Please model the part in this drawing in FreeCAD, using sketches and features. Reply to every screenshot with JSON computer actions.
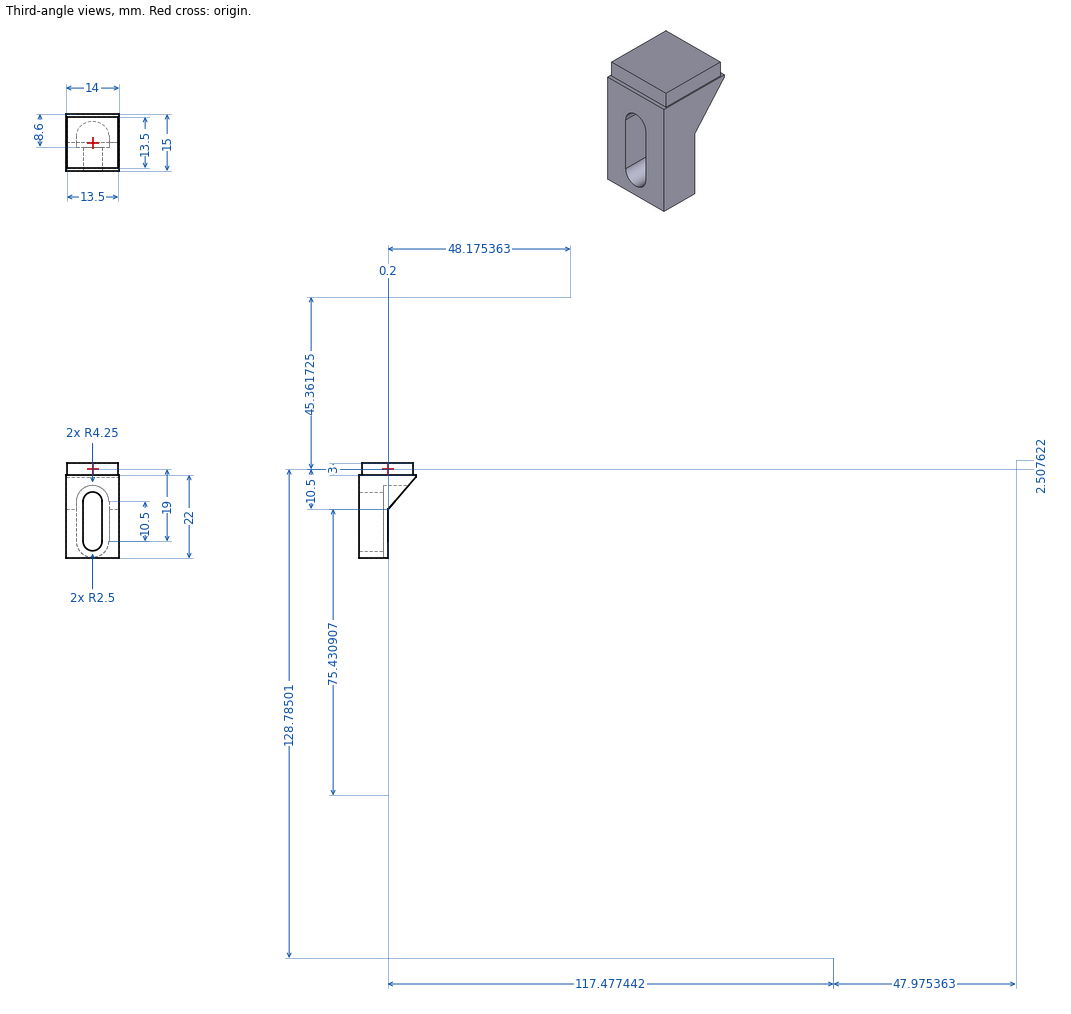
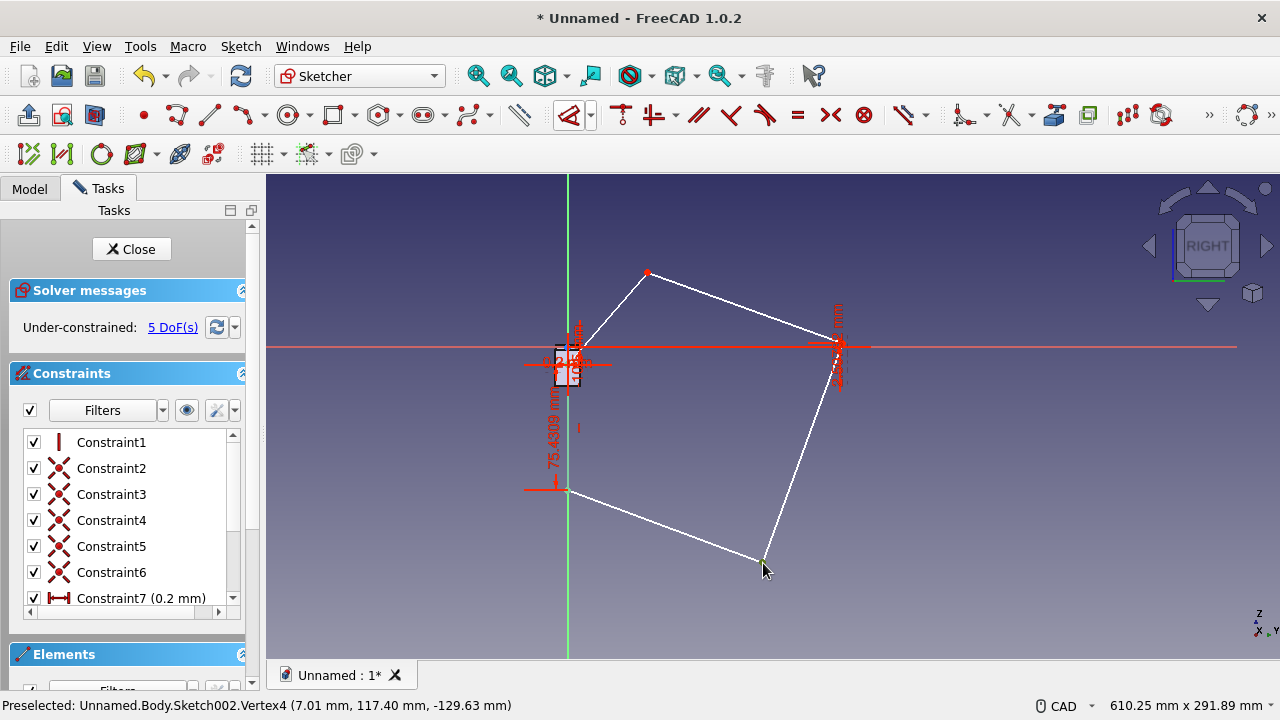
{"action": "key", "text": "i"}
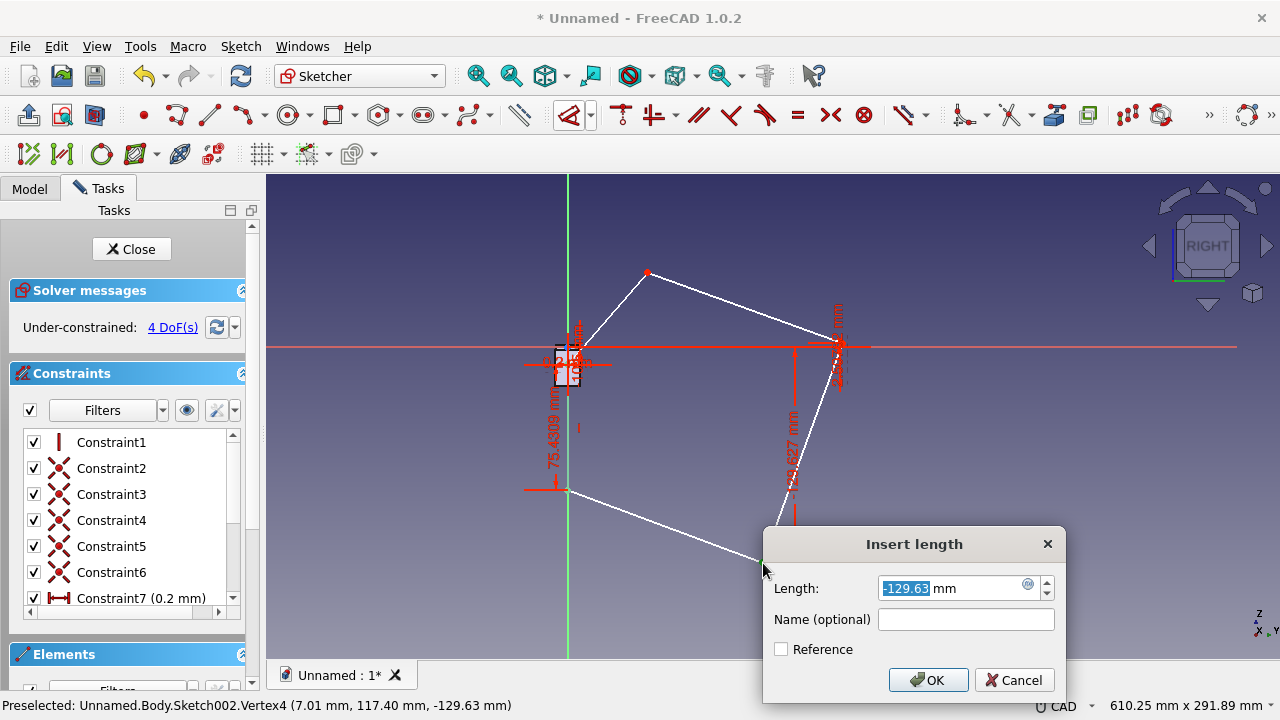
{"action": "type", "text": "-128.78501"}
{"action": "key", "text": "Return"}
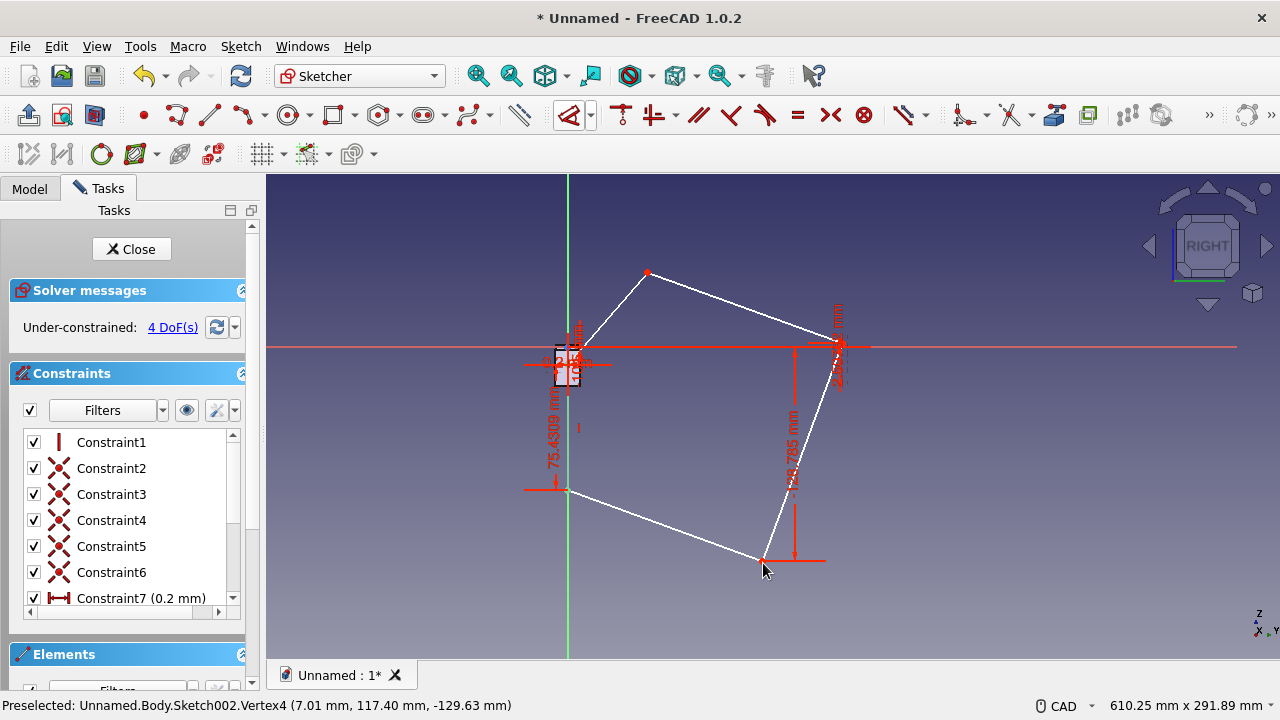
{"action": "left_click", "coordinate": [648, 273]}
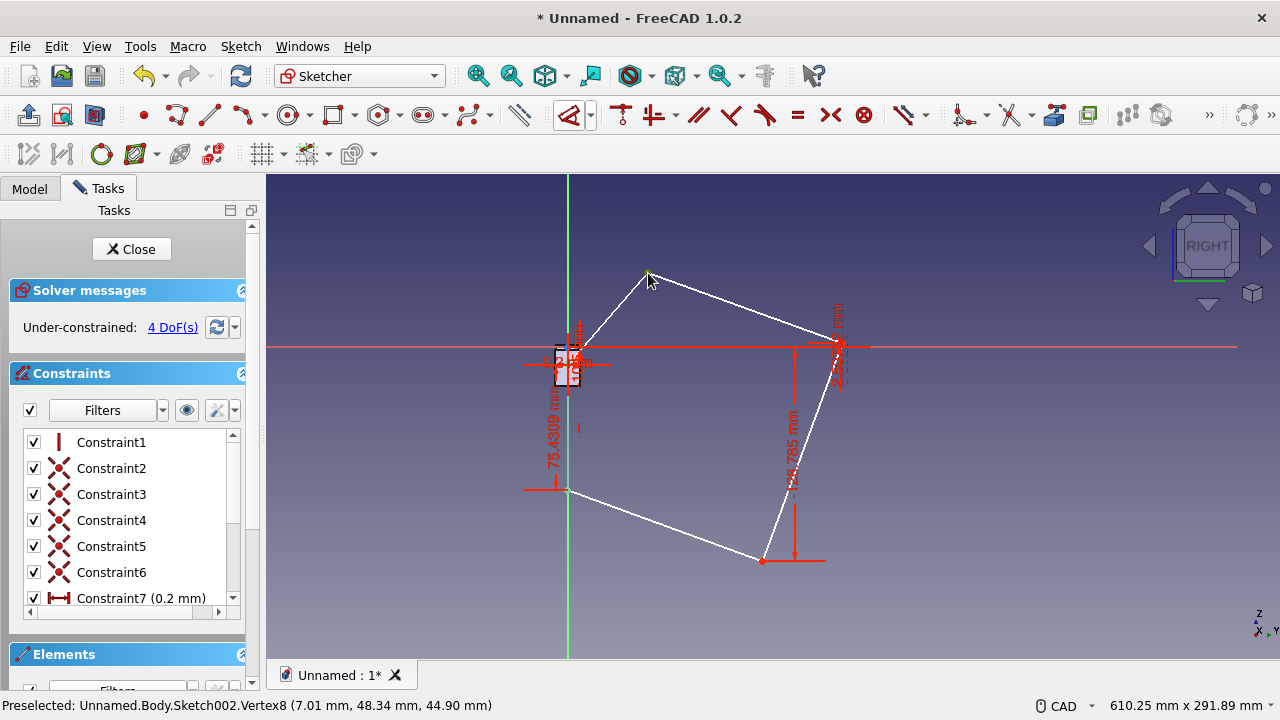
{"action": "key", "text": "l"}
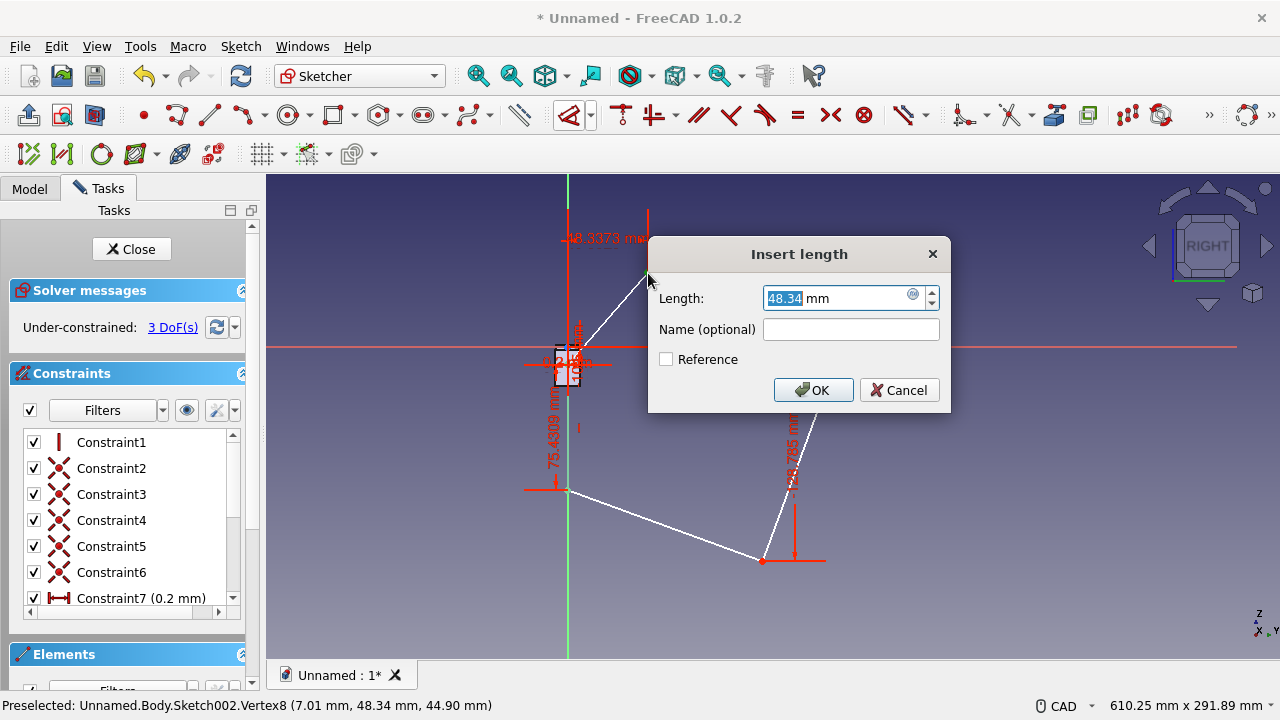
{"action": "type", "text": "48.175363"}
{"action": "key", "text": "Return"}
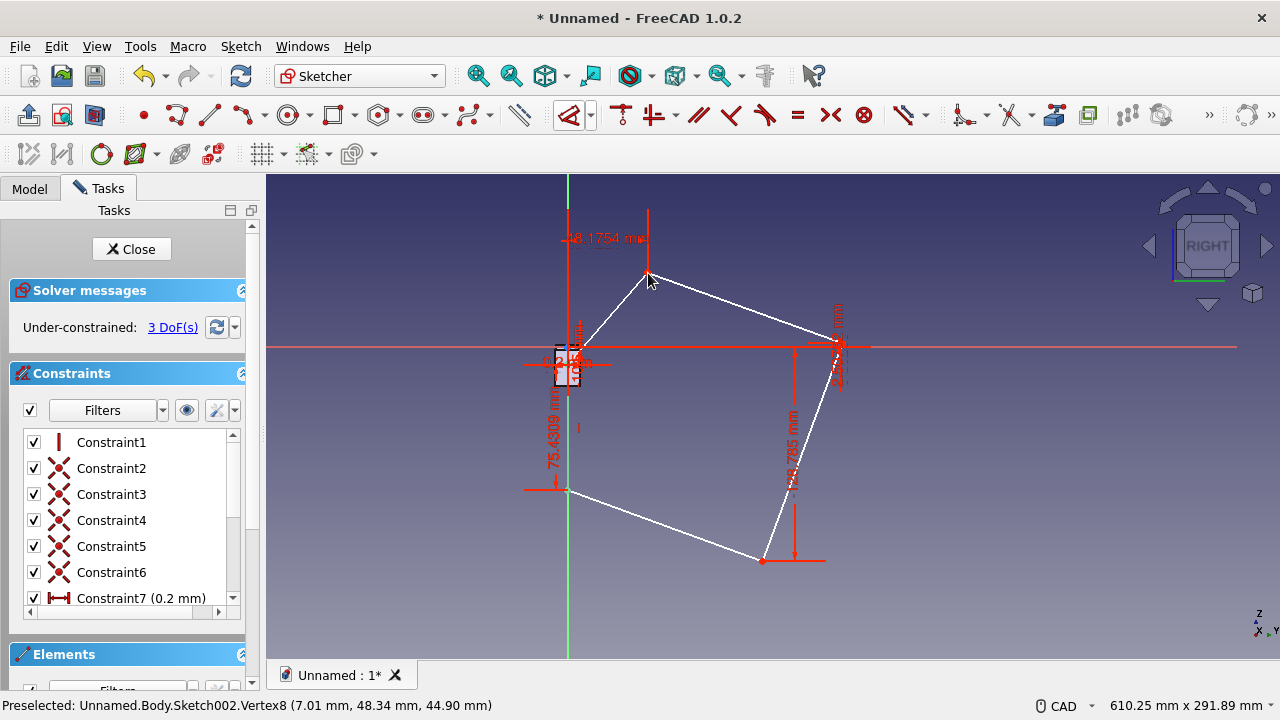
{"action": "left_click", "coordinate": [648, 273]}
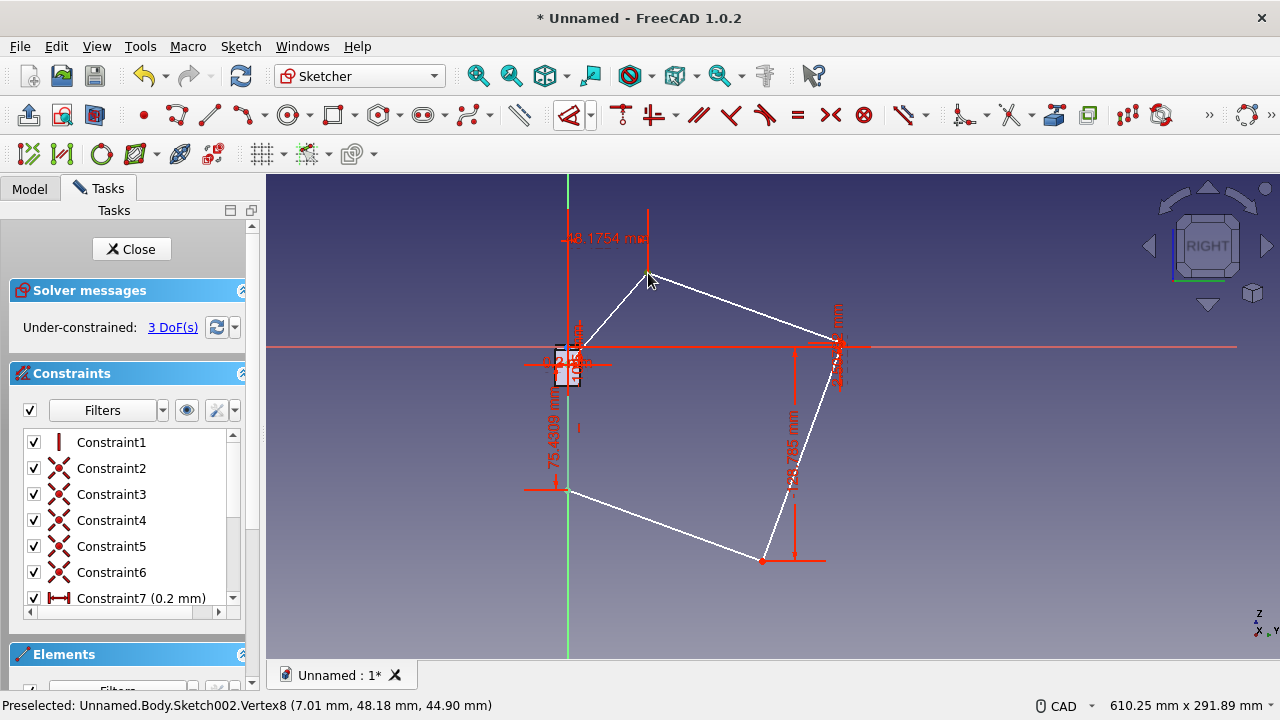
{"action": "key", "text": "i"}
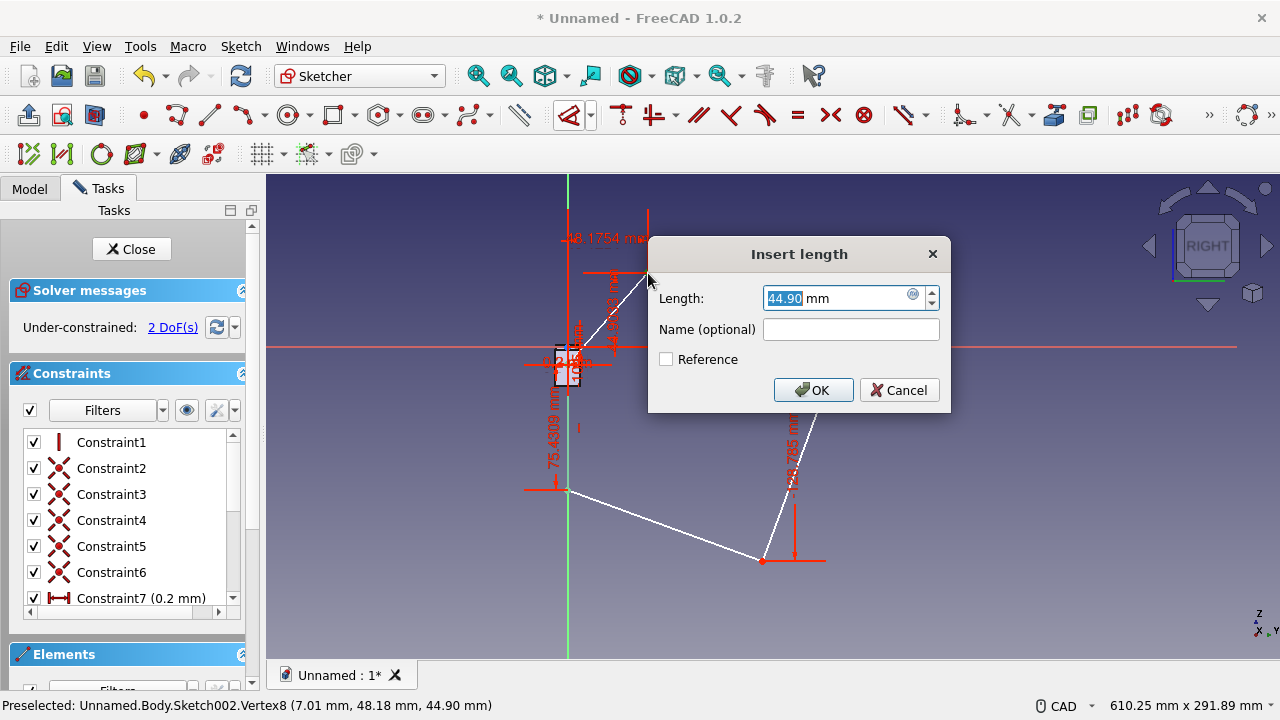
{"action": "type", "text": "45.361725"}
{"action": "key", "text": "Return"}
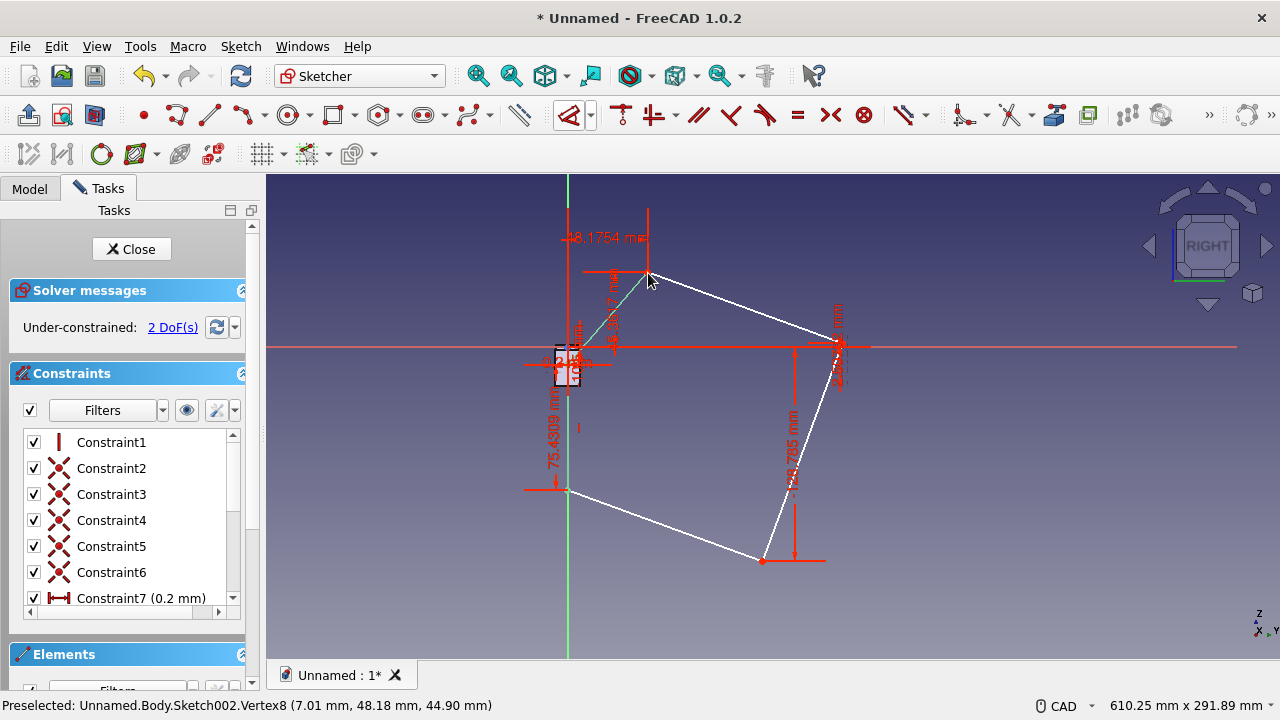
{"action": "left_click", "coordinate": [819, 409]}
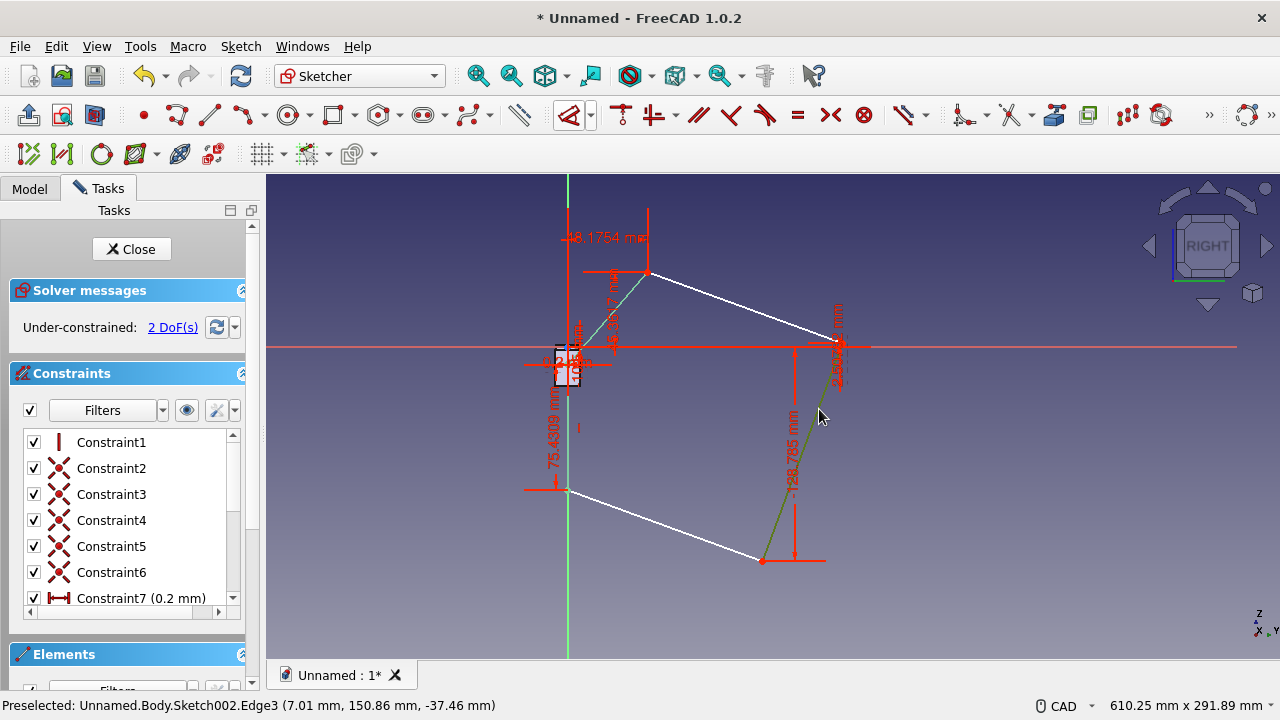
{"action": "key", "text": "l"}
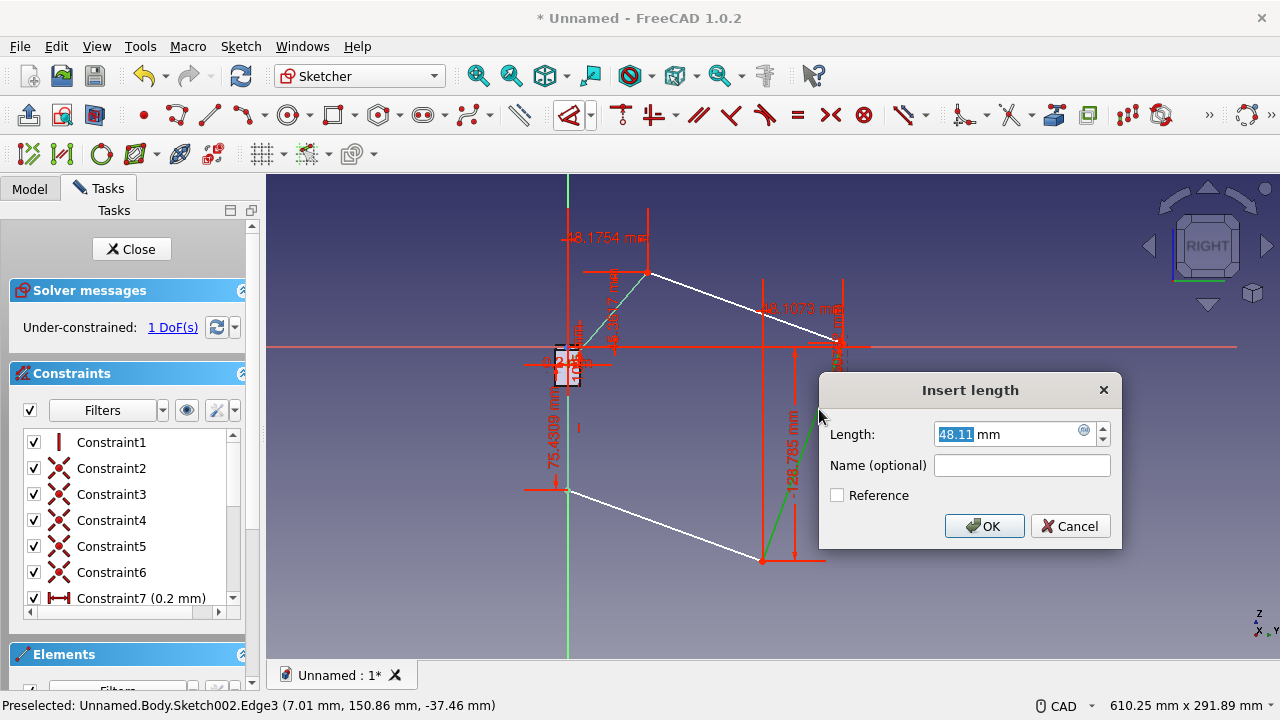
{"action": "type", "text": "47.975363"}
{"action": "key", "text": "Return"}